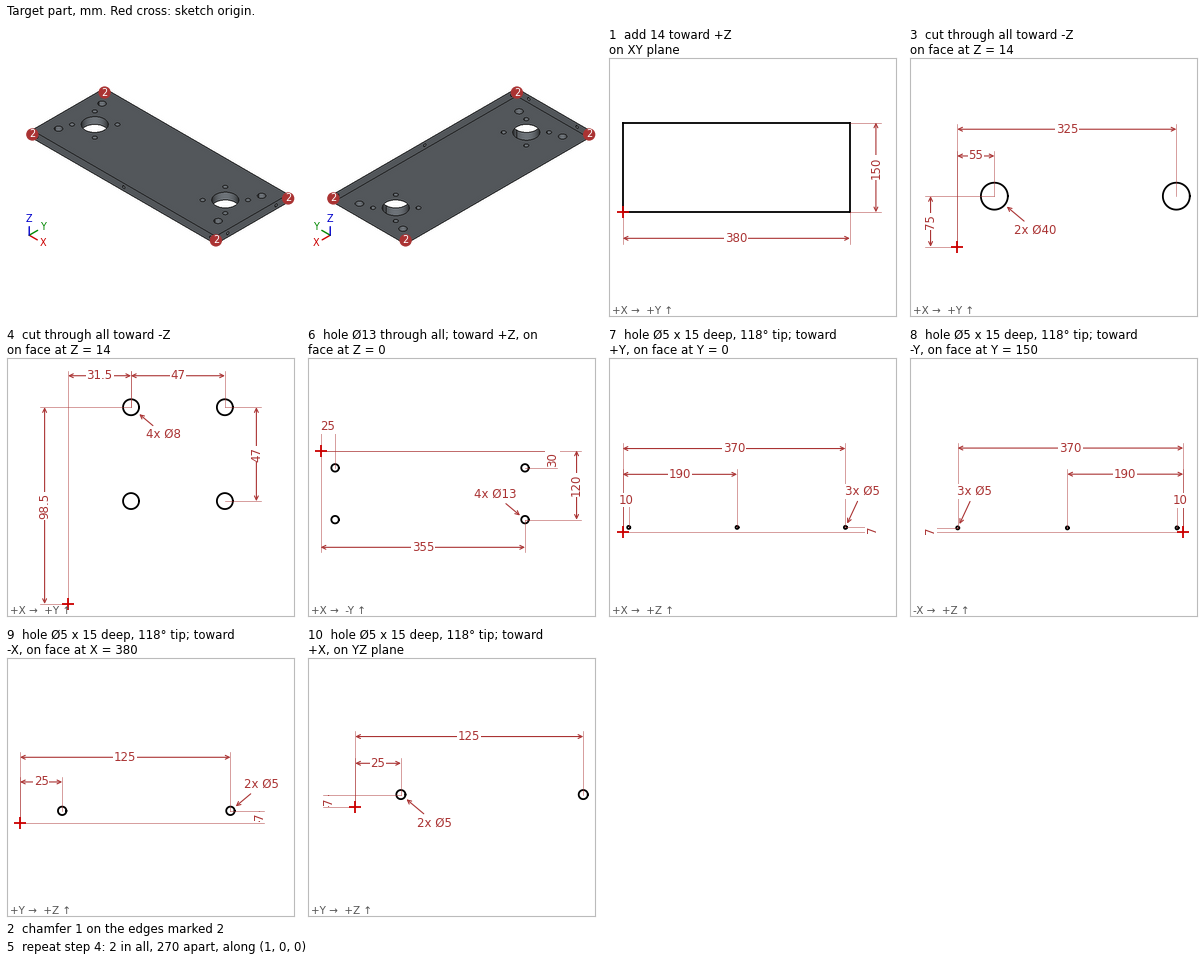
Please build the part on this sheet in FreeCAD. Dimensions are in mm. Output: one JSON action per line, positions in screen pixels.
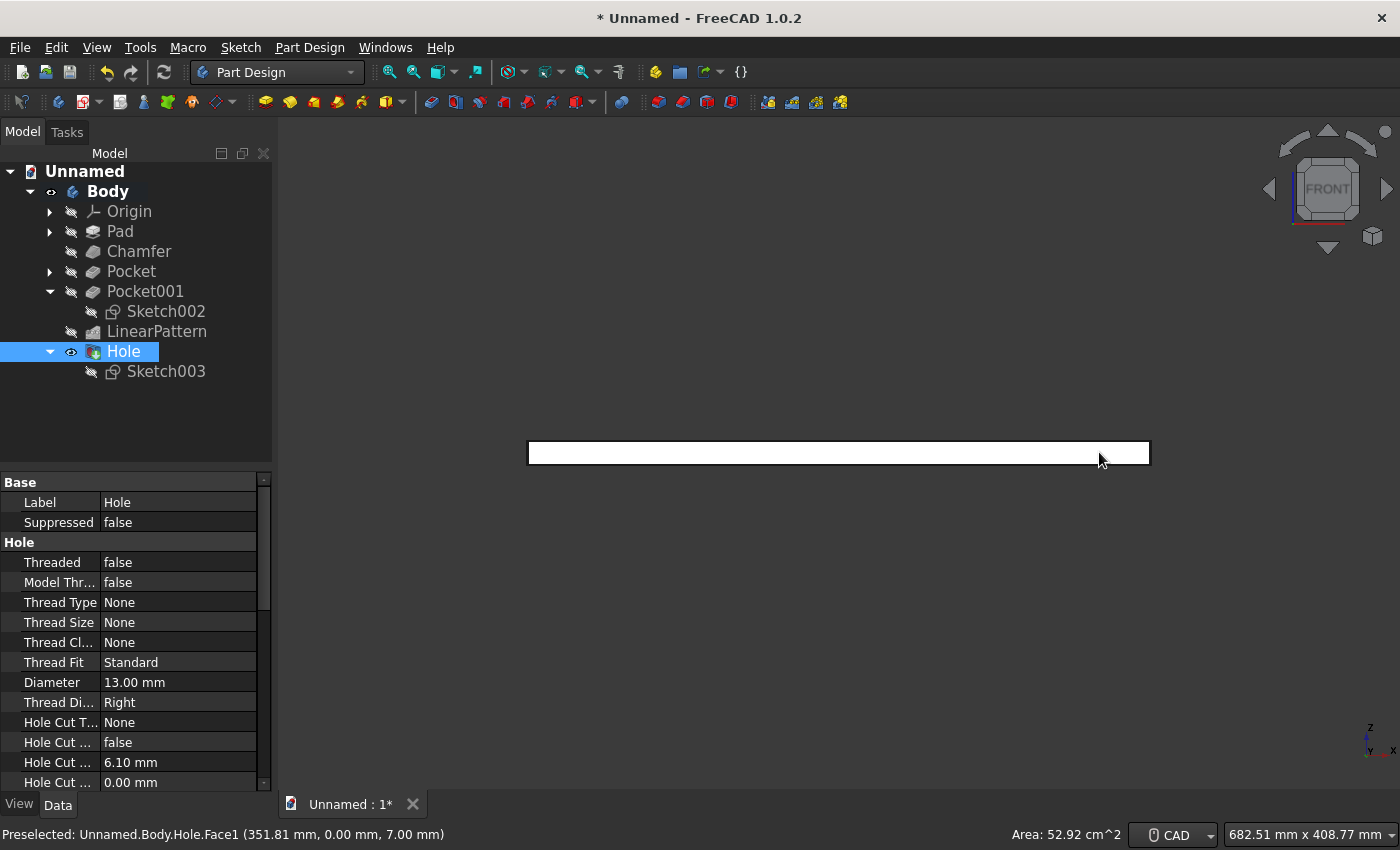
{"action": "left_click", "coordinate": [84, 102]}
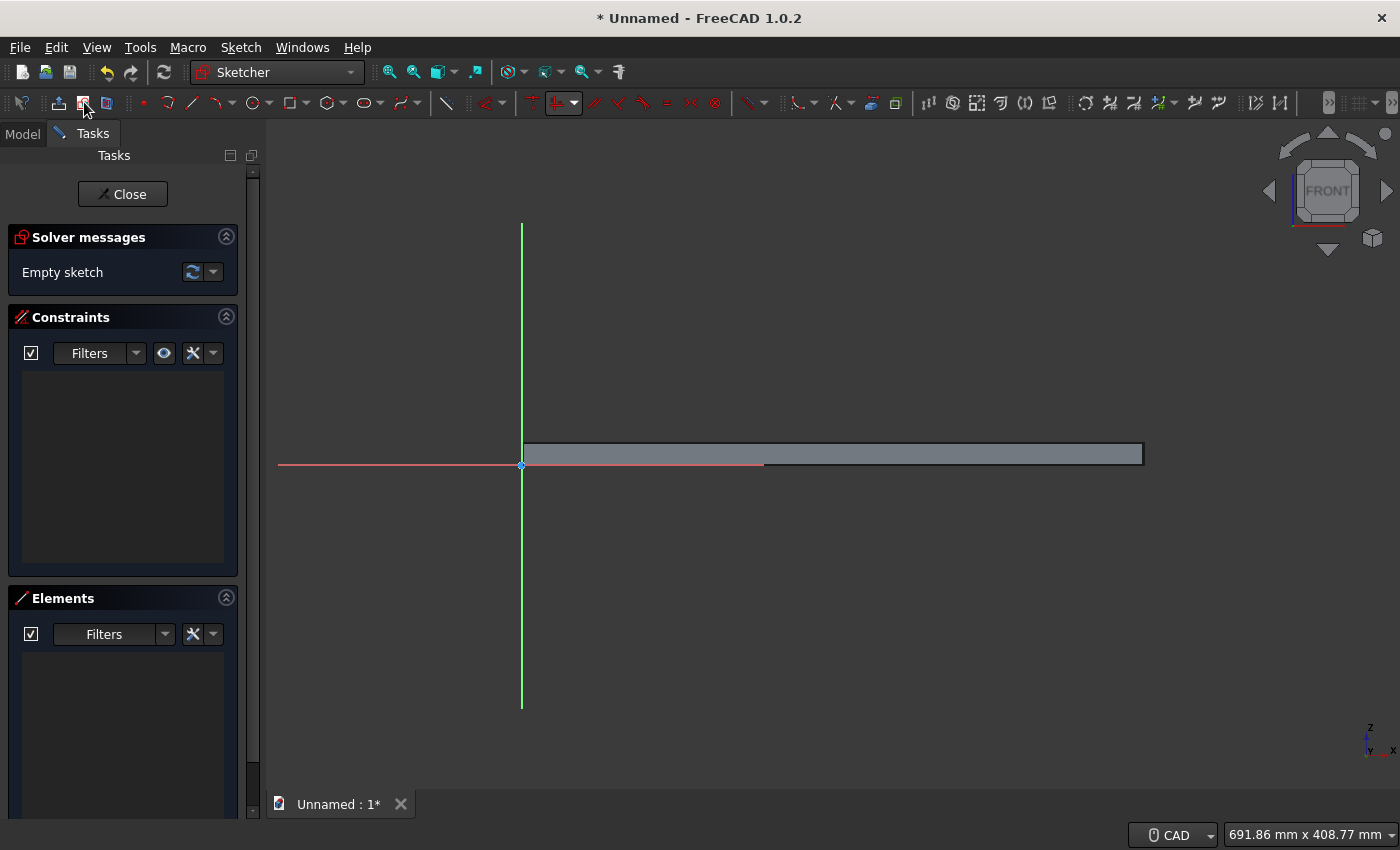
{"action": "key", "text": "g c"}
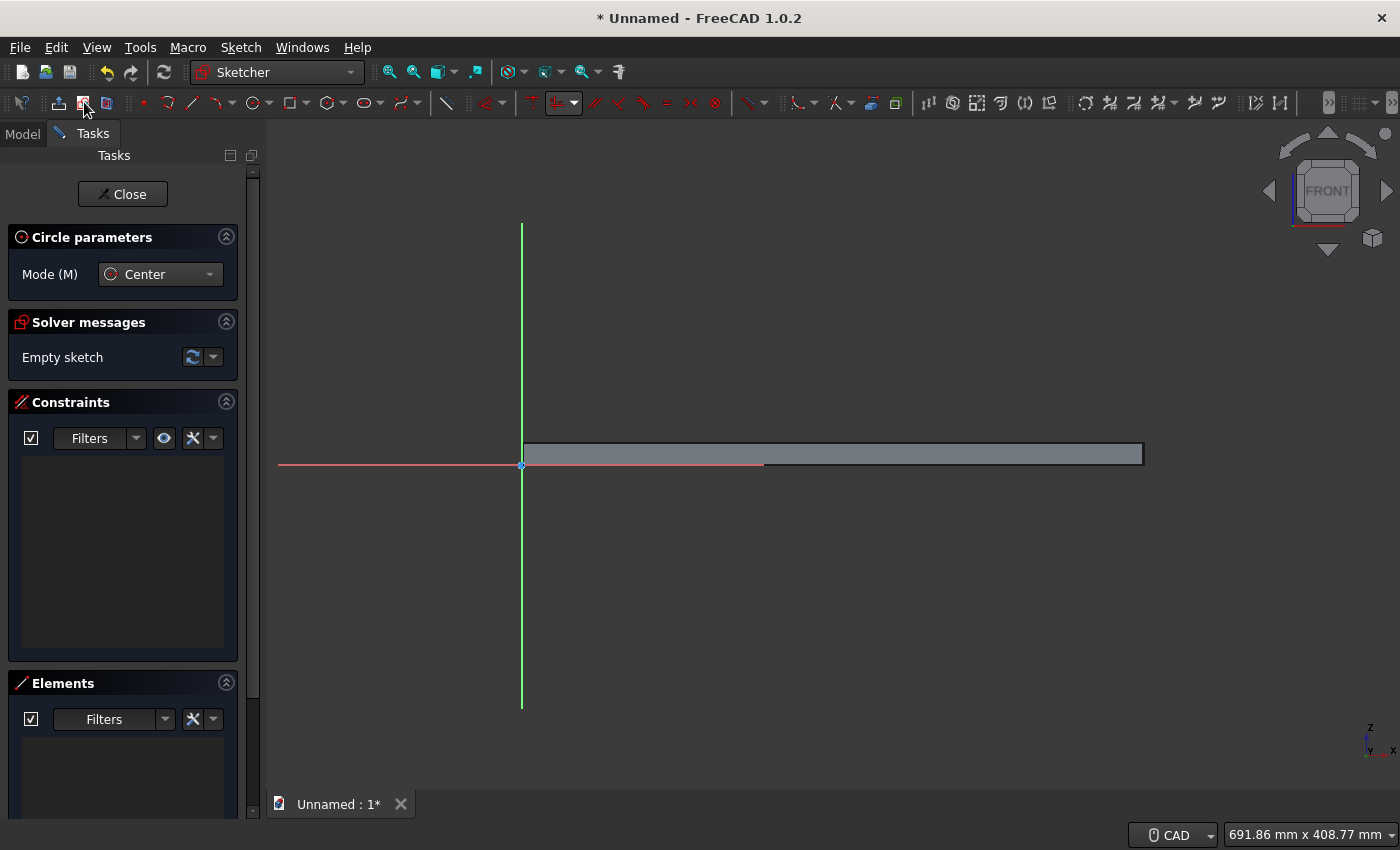
{"action": "scroll", "coordinate": [1128, 454], "scroll_direction": "up", "scroll_amount": 9}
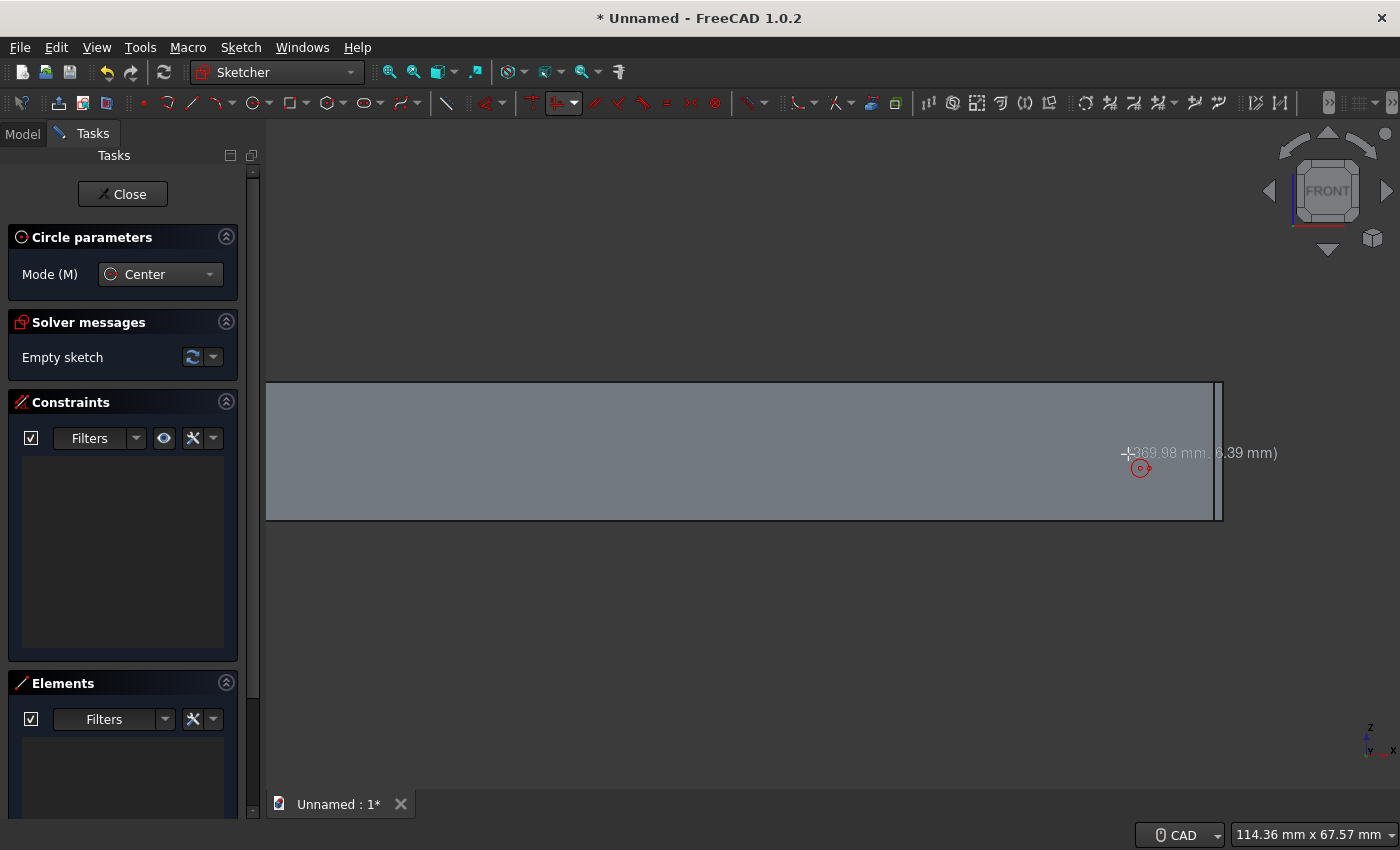
{"action": "scroll", "coordinate": [1054, 450], "scroll_direction": "down", "scroll_amount": 9}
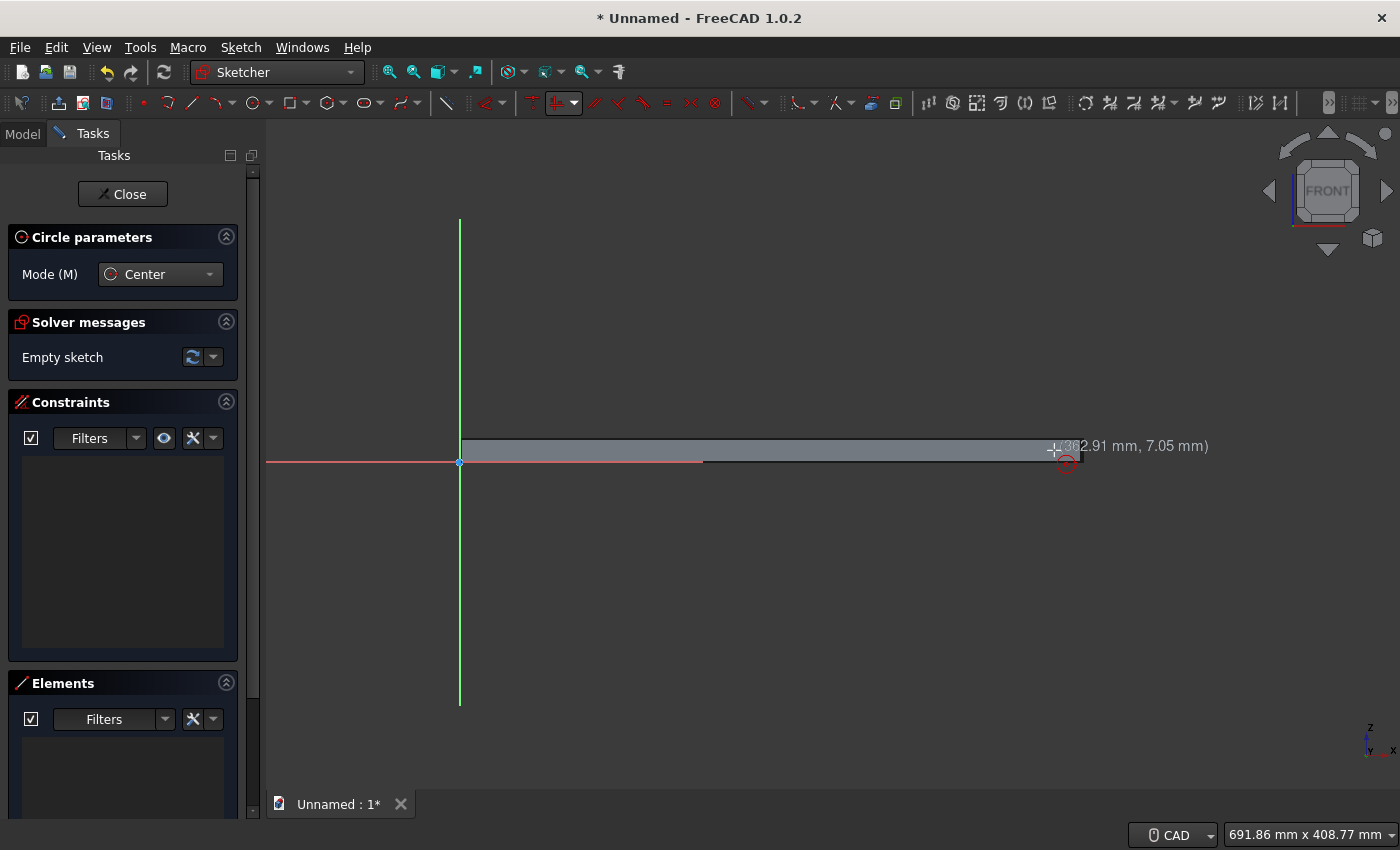
{"action": "scroll", "coordinate": [1066, 451], "scroll_direction": "up", "scroll_amount": 2}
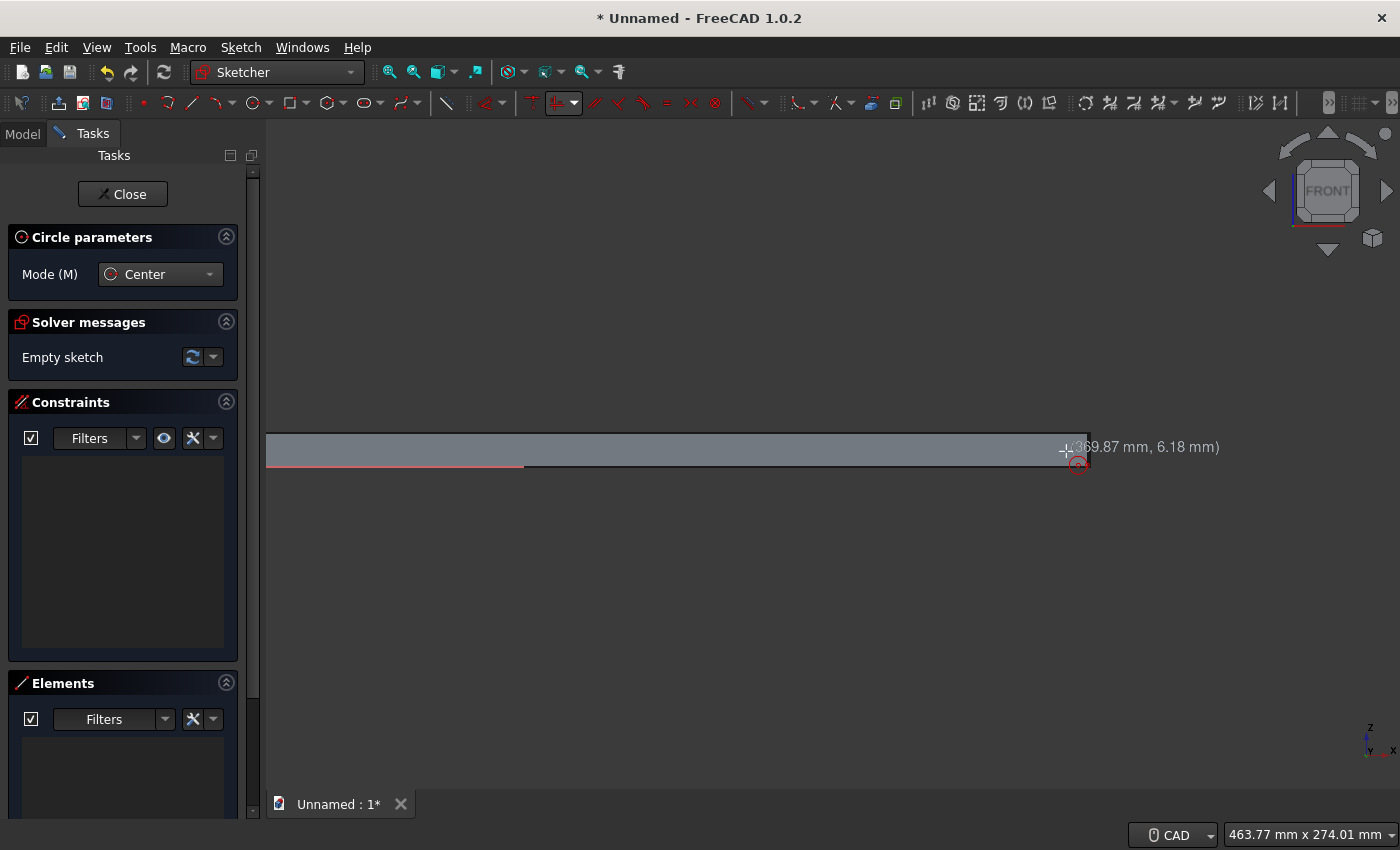
{"action": "left_click", "coordinate": [1066, 450]}
{"action": "mouse_move", "coordinate": [1070, 446]}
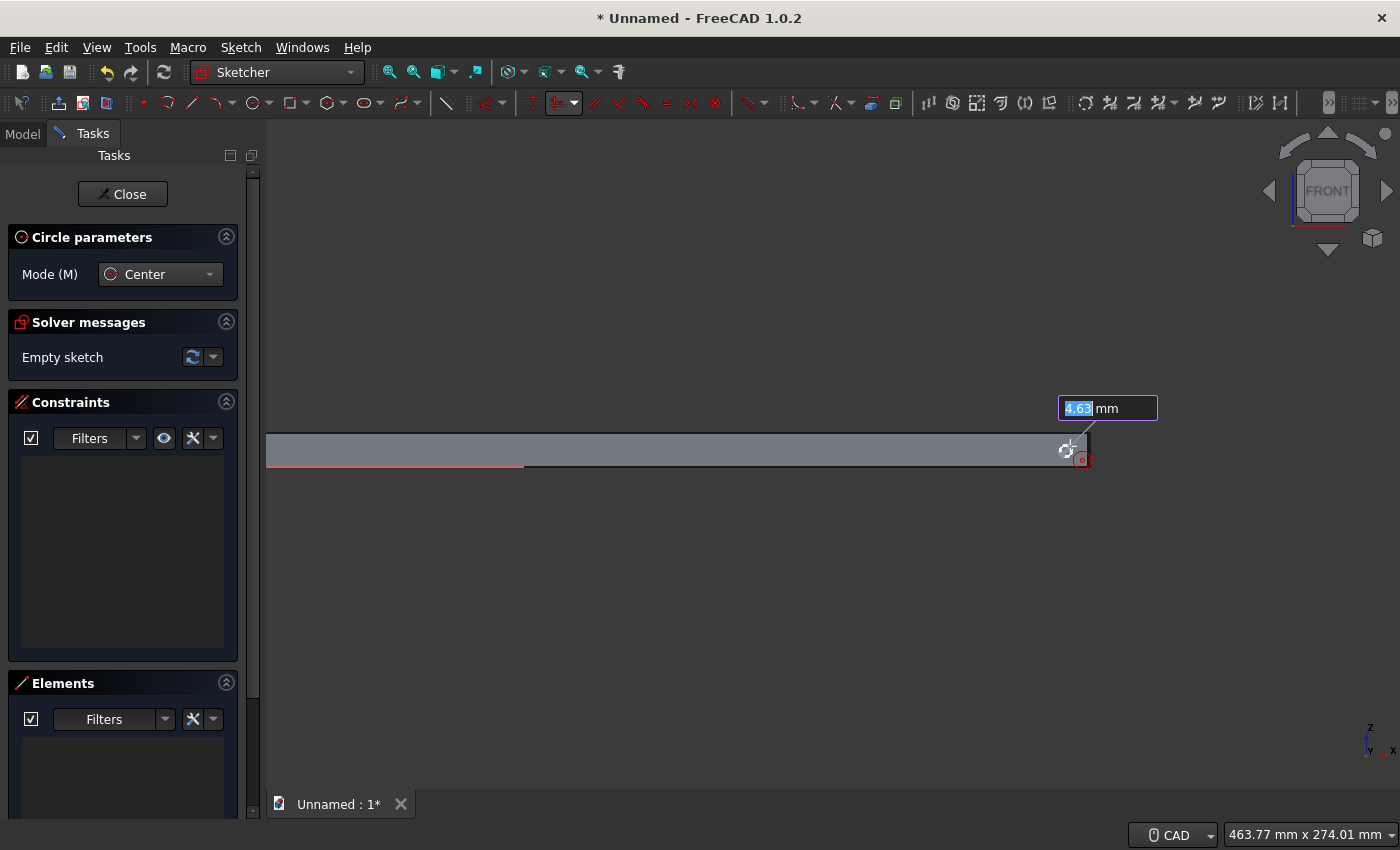
{"action": "type", "text": "5"}
{"action": "key", "text": "Return"}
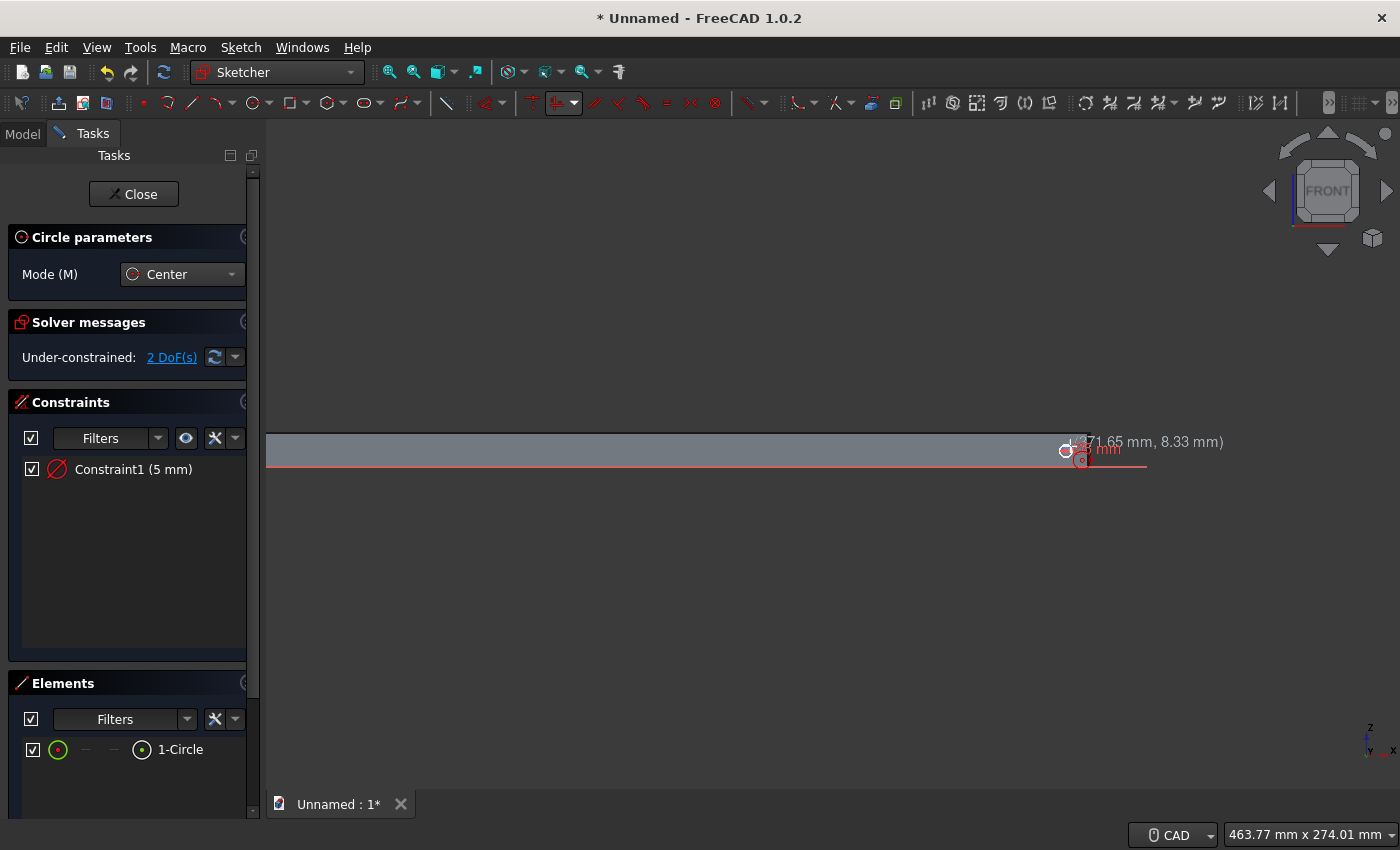
{"action": "scroll", "coordinate": [626, 450], "scroll_direction": "up", "scroll_amount": 7}